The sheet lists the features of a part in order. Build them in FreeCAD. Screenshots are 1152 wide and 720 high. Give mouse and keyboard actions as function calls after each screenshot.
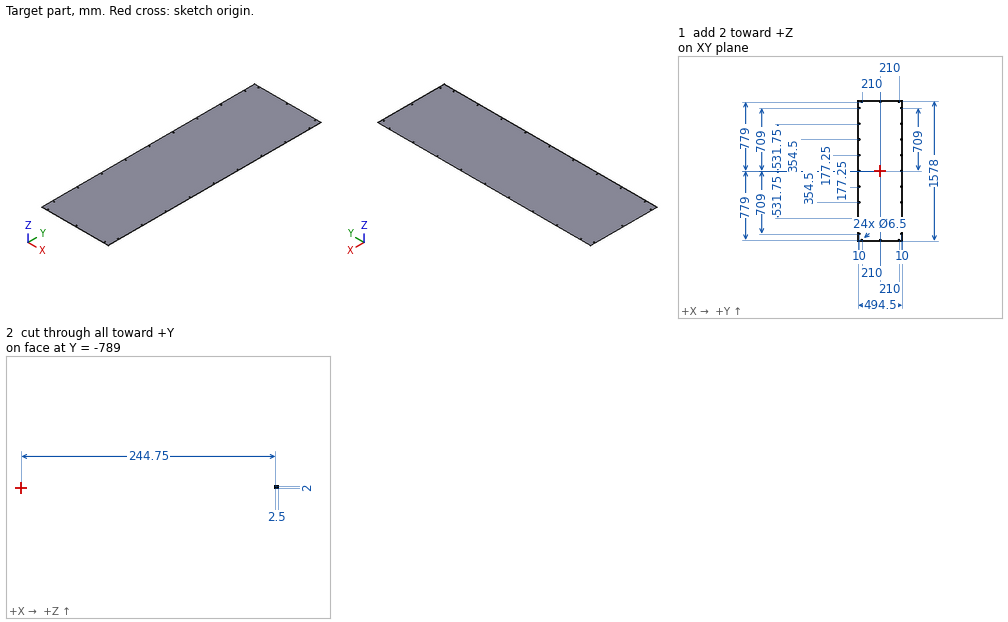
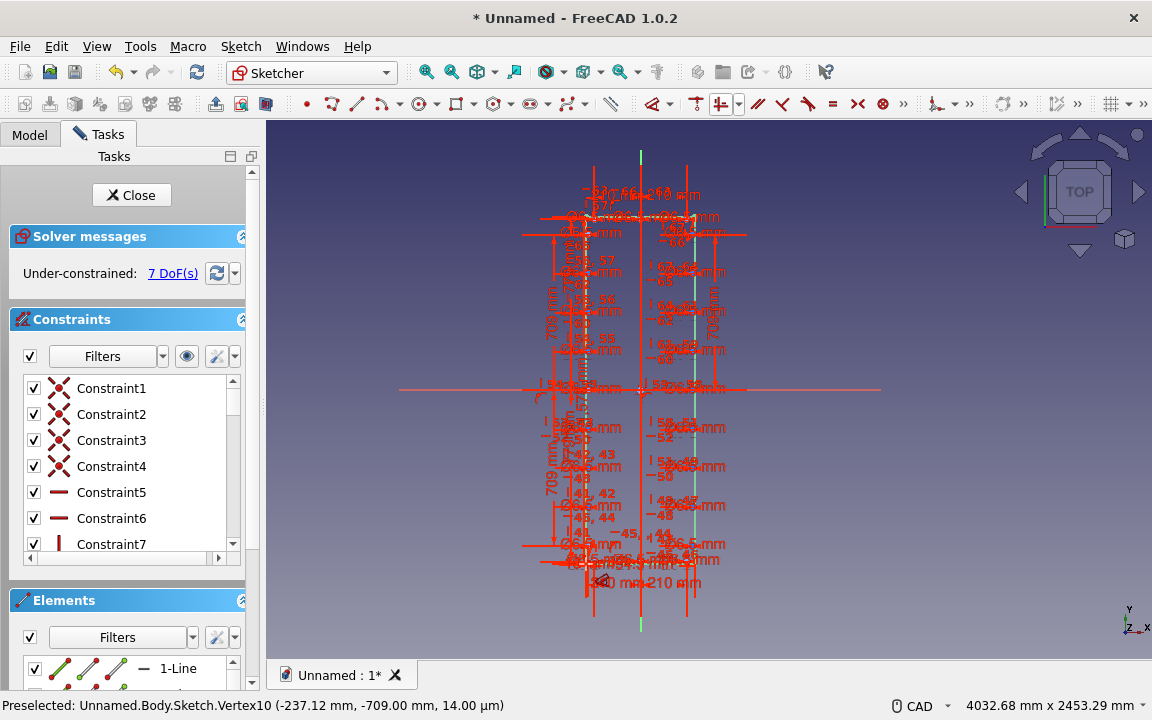
scroll(695, 564, up, 15)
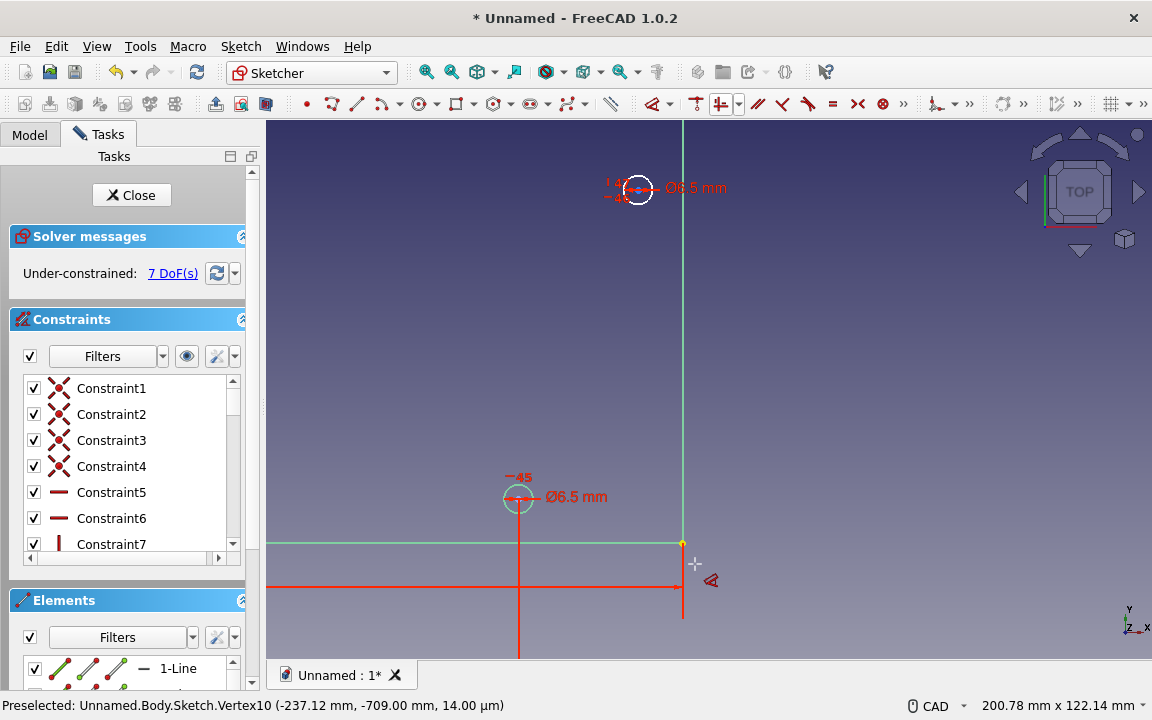
click(683, 543)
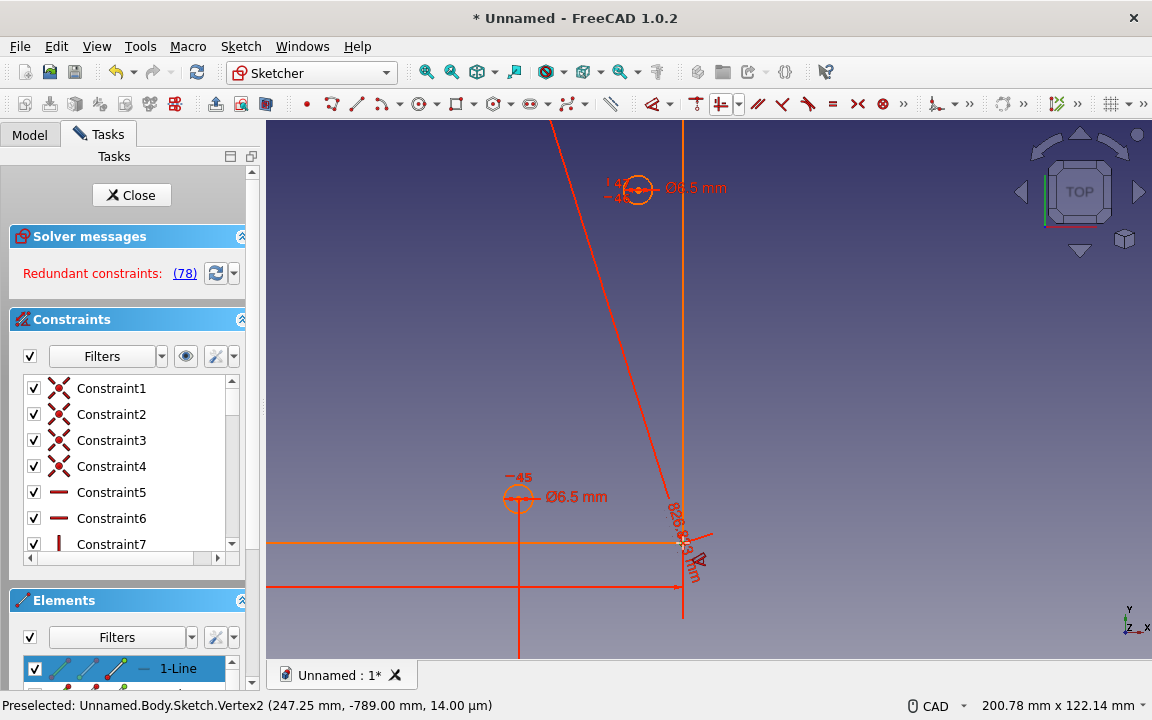
click(638, 190)
click(660, 577)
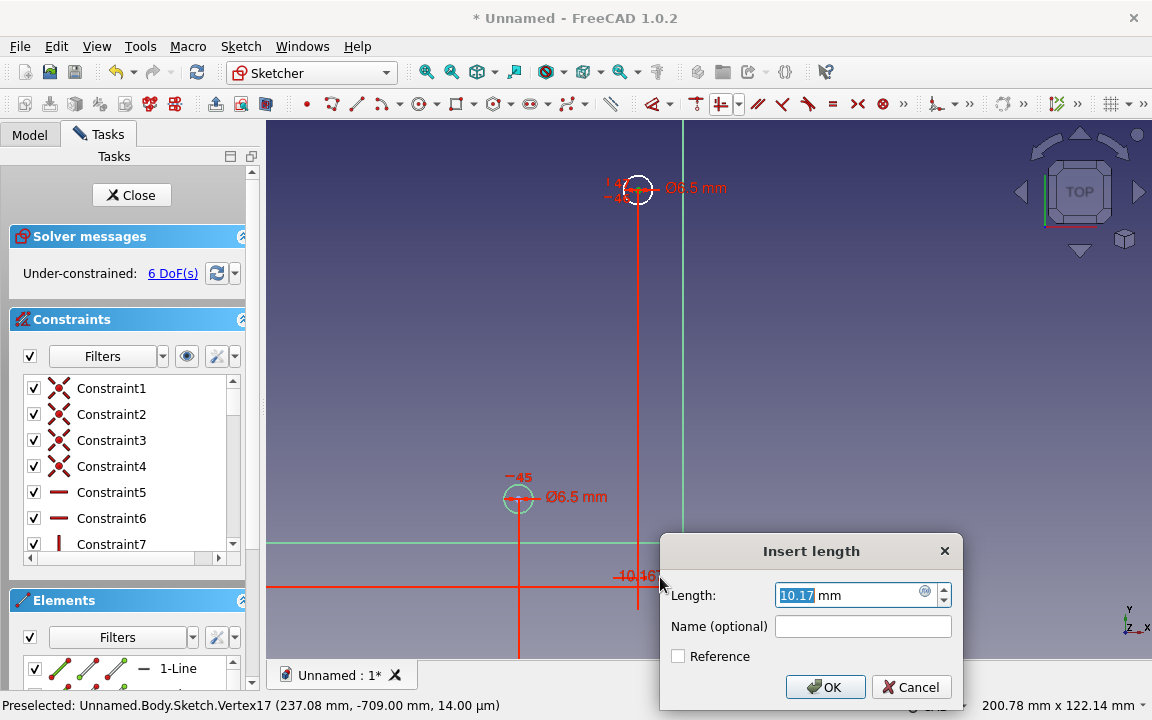
text(10)
key(Return)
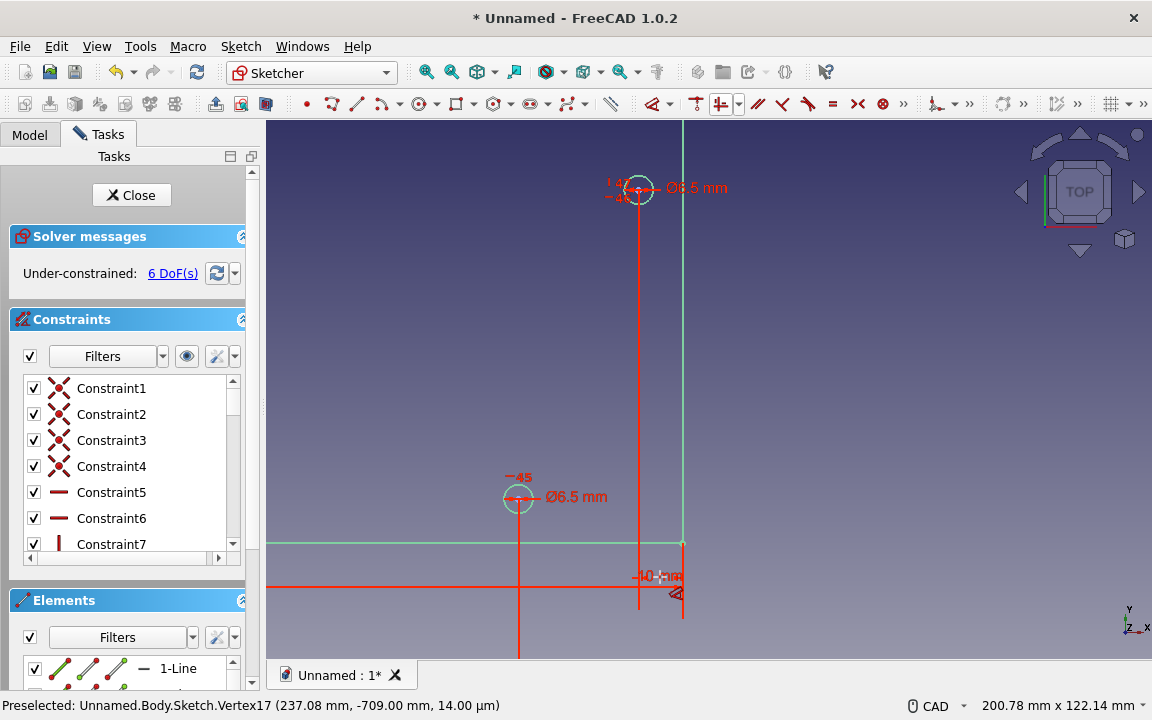
scroll(695, 564, down, 15)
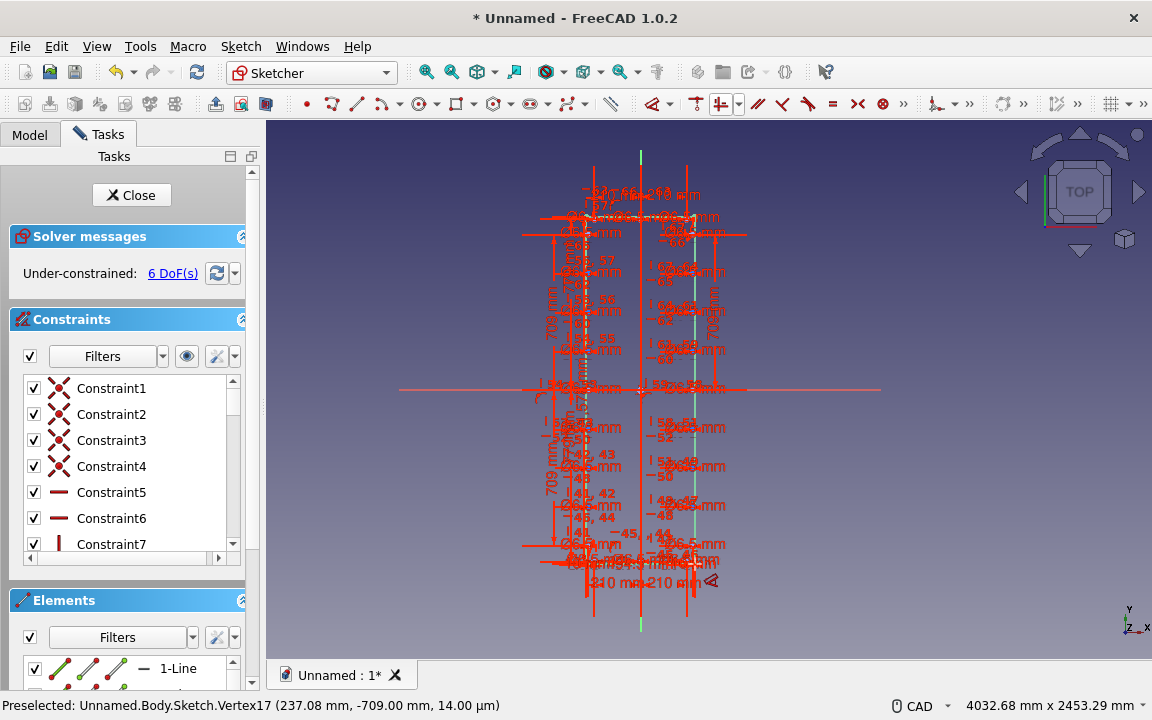
click(588, 468)
click(554, 411)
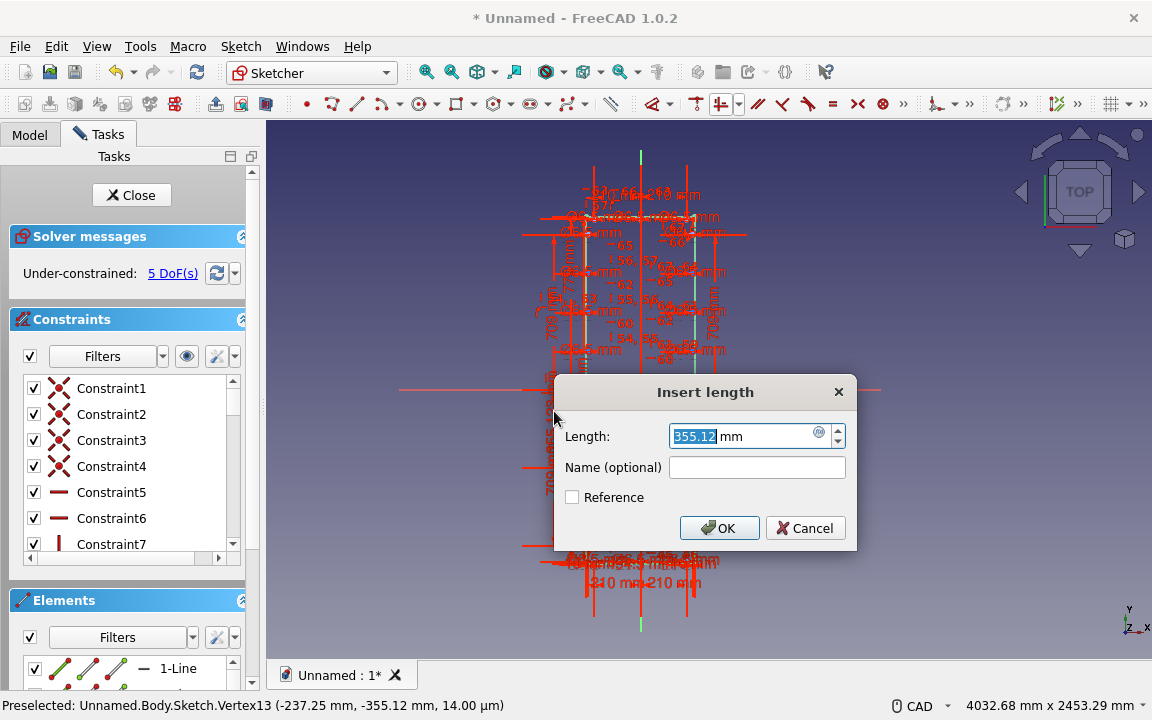
text(354.5)
key(Return)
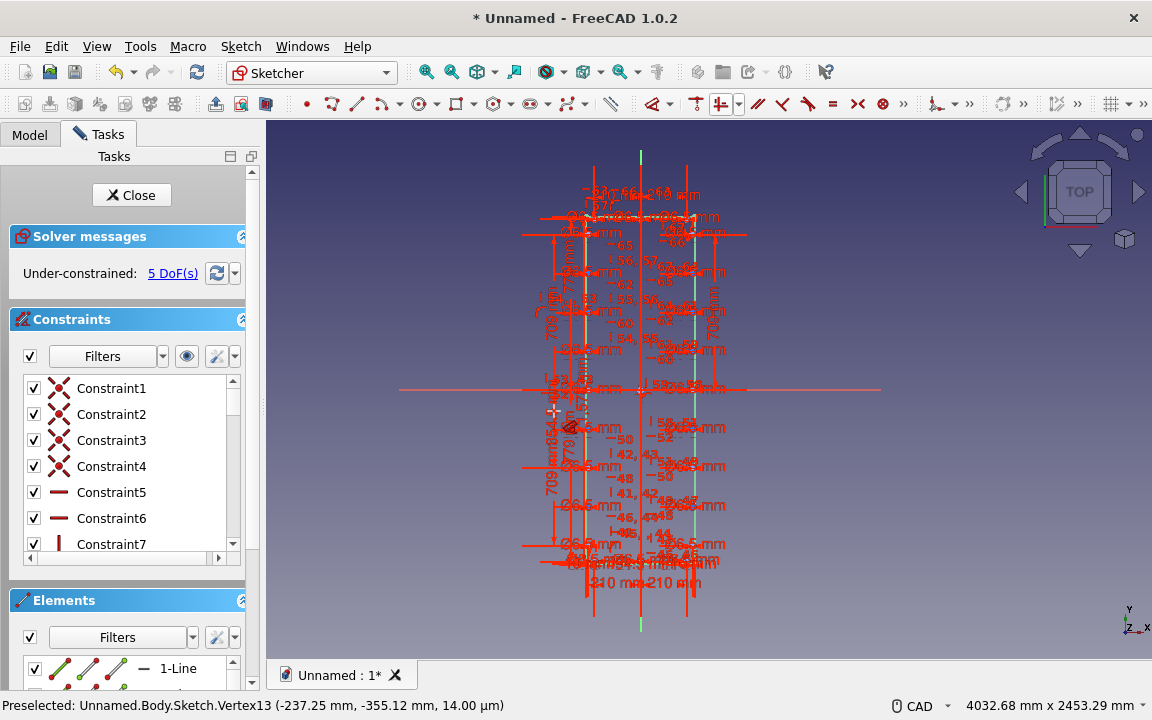
click(588, 313)
click(554, 352)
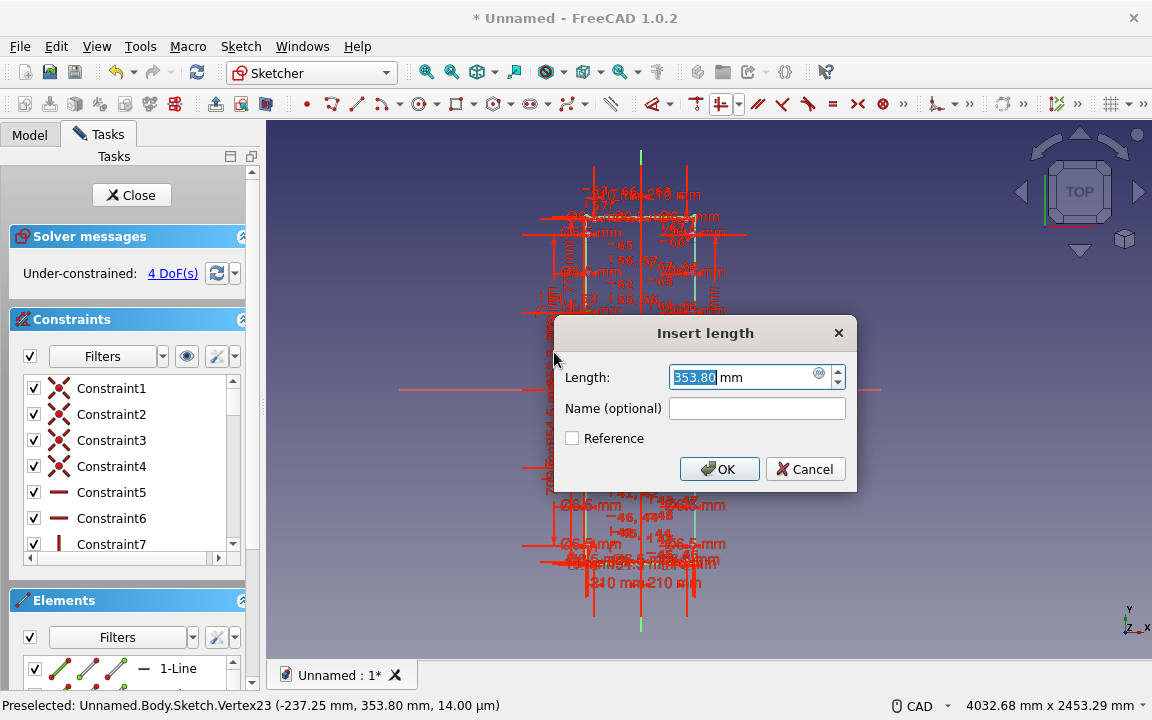
text(354.5)
key(Return)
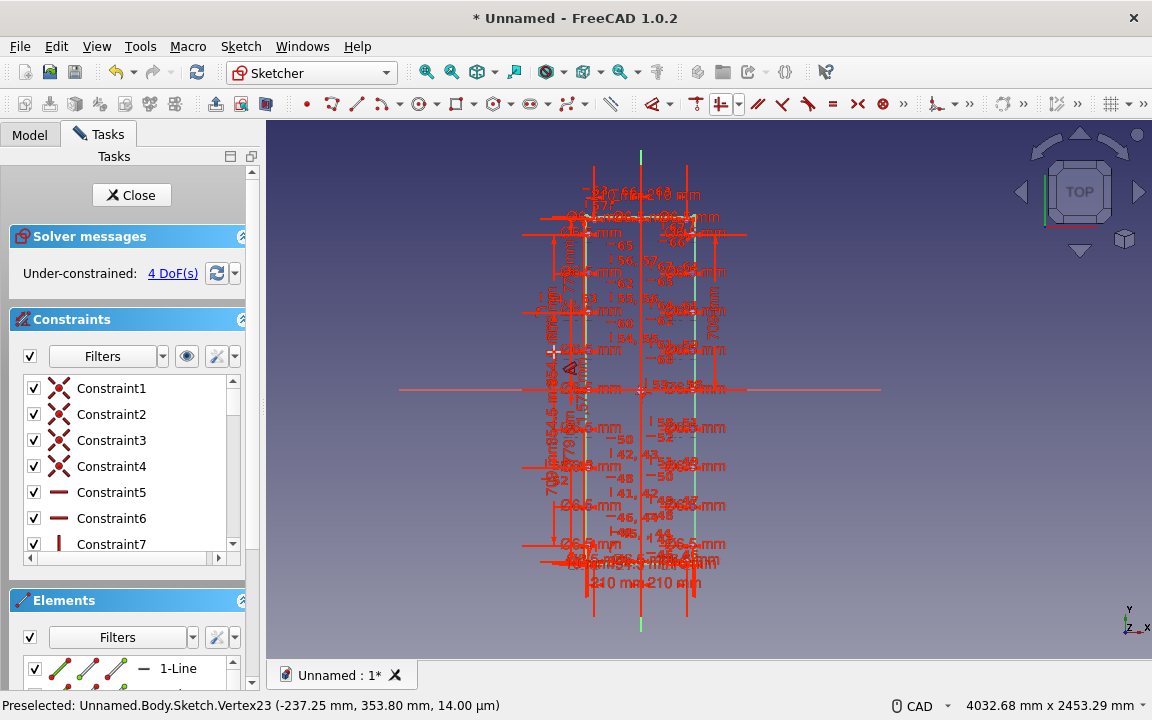
click(588, 507)
click(554, 490)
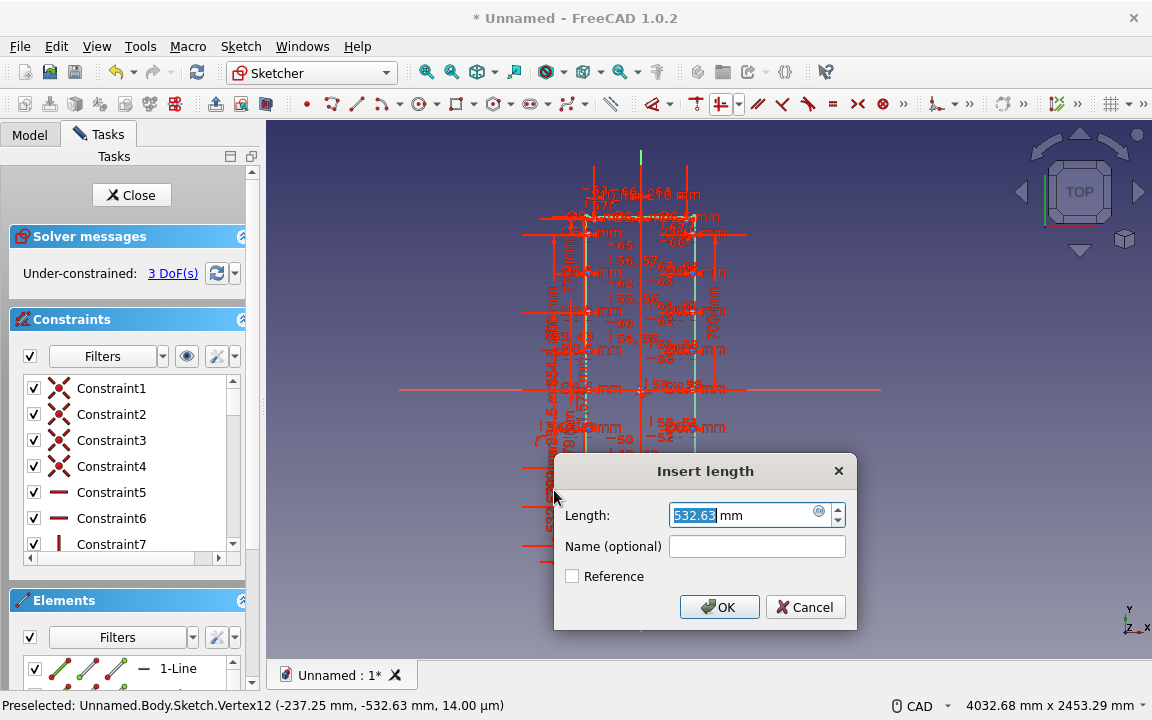
text(531.75)
key(Return)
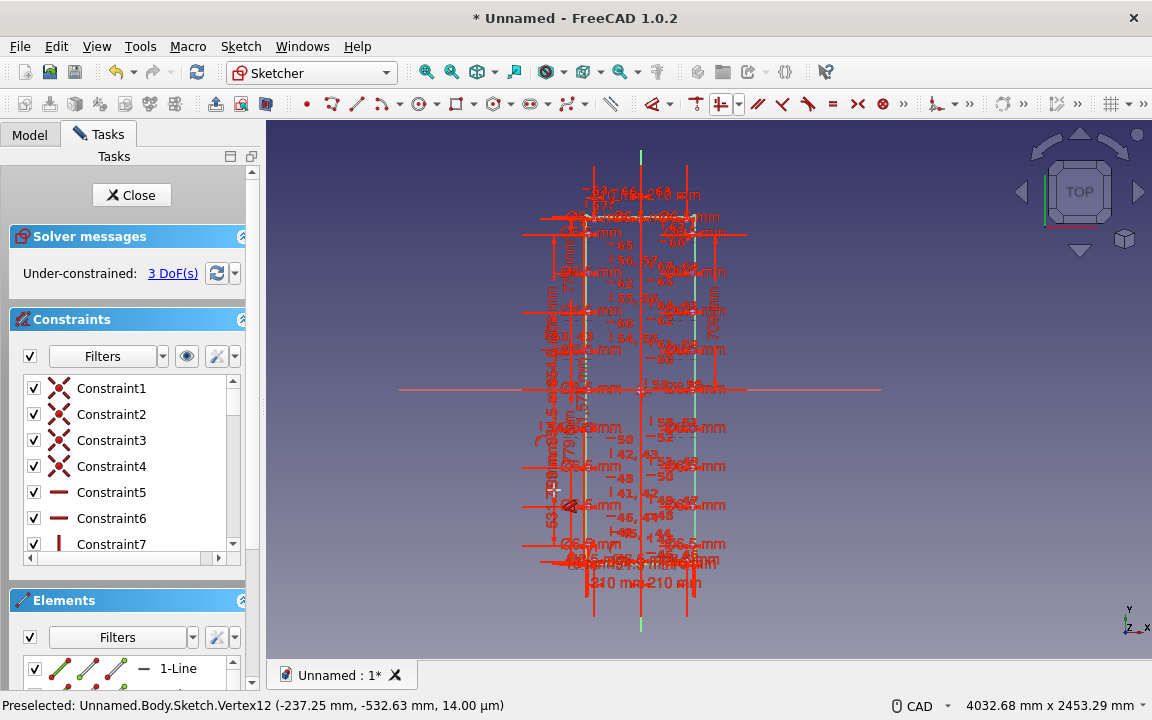
click(588, 430)
click(675, 410)